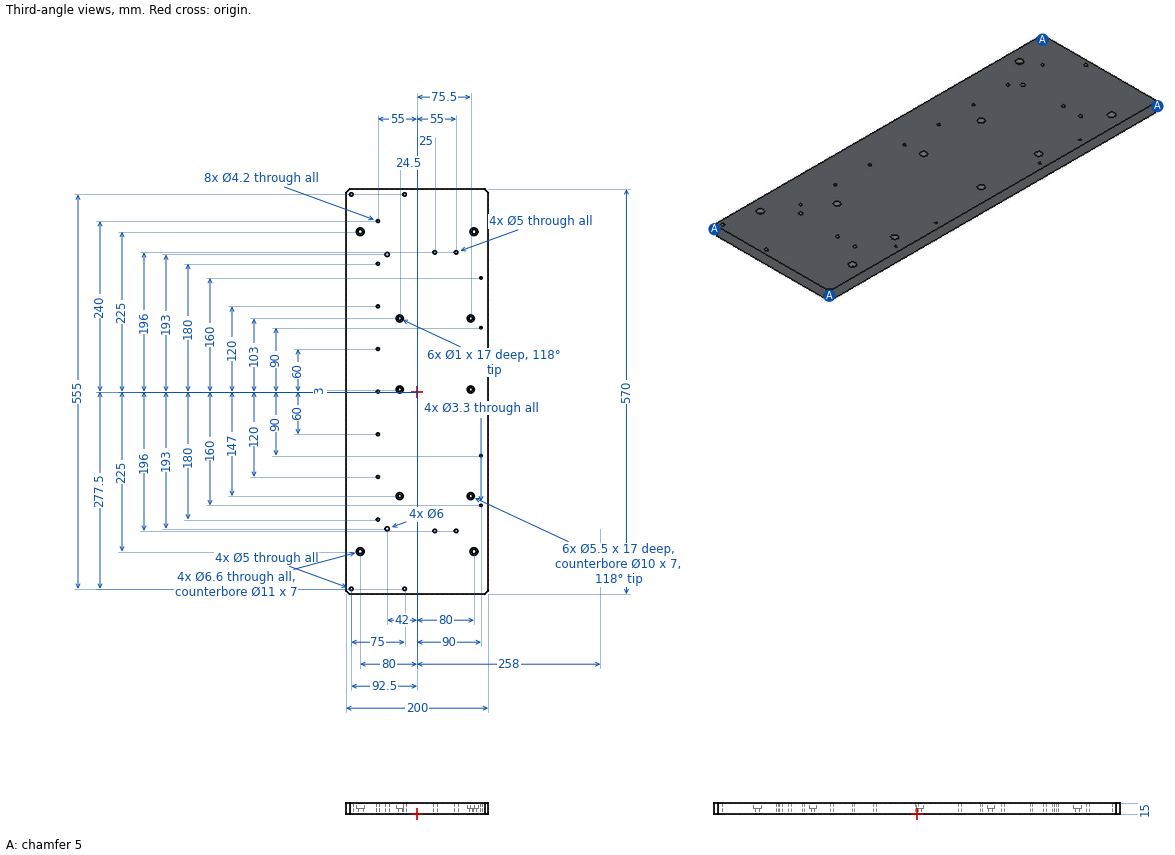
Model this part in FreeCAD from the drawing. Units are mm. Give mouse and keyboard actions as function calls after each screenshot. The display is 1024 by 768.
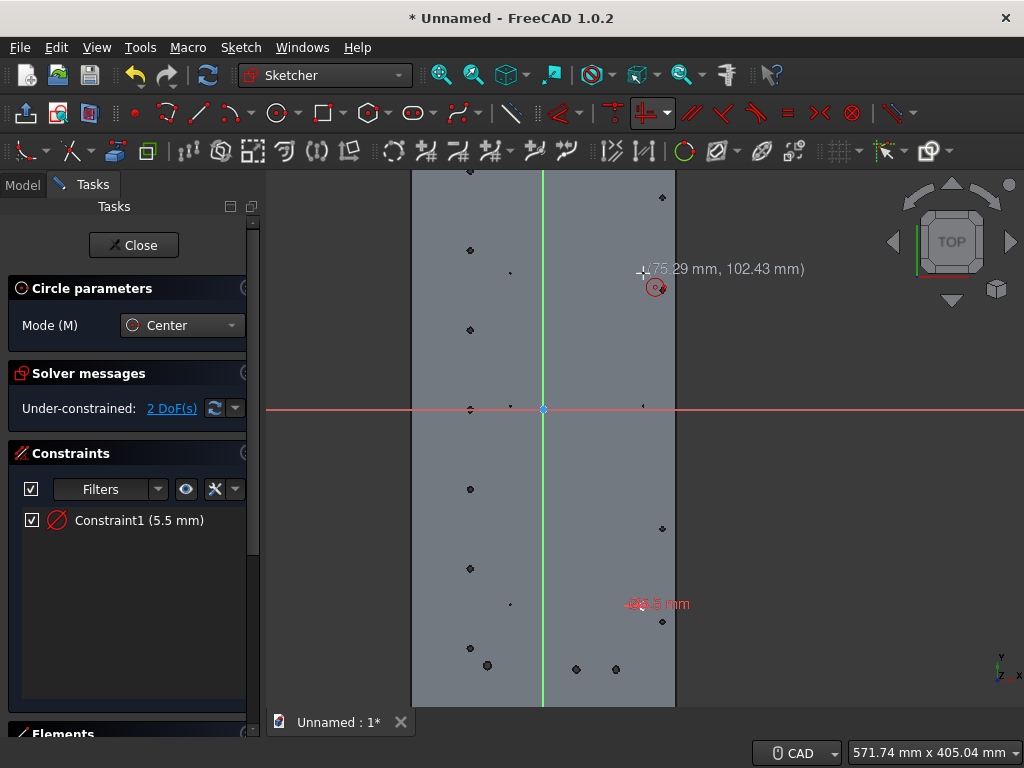
click(643, 273)
move(646, 271)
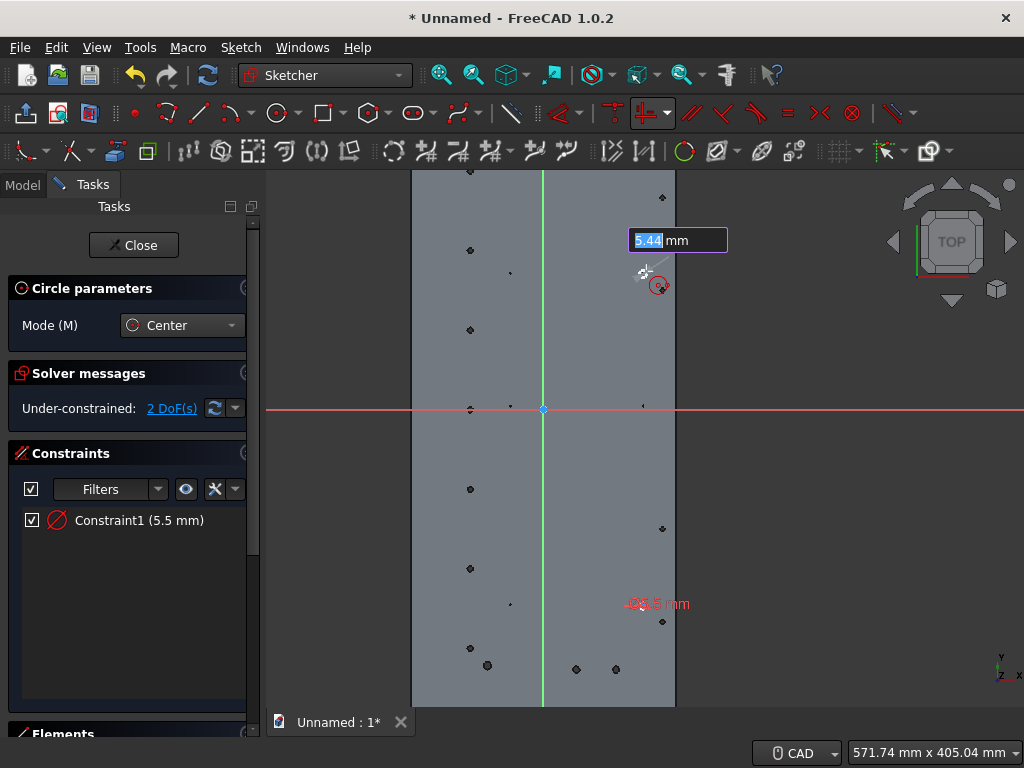
text(5.5)
key(Return)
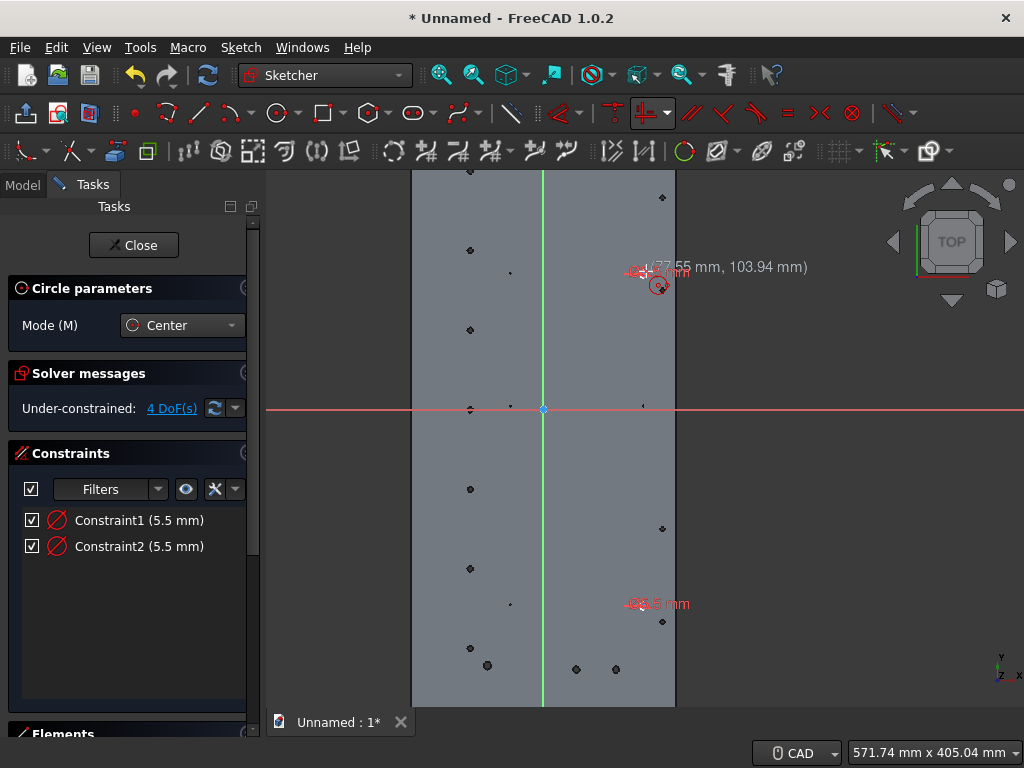
scroll(643, 406, up, 10)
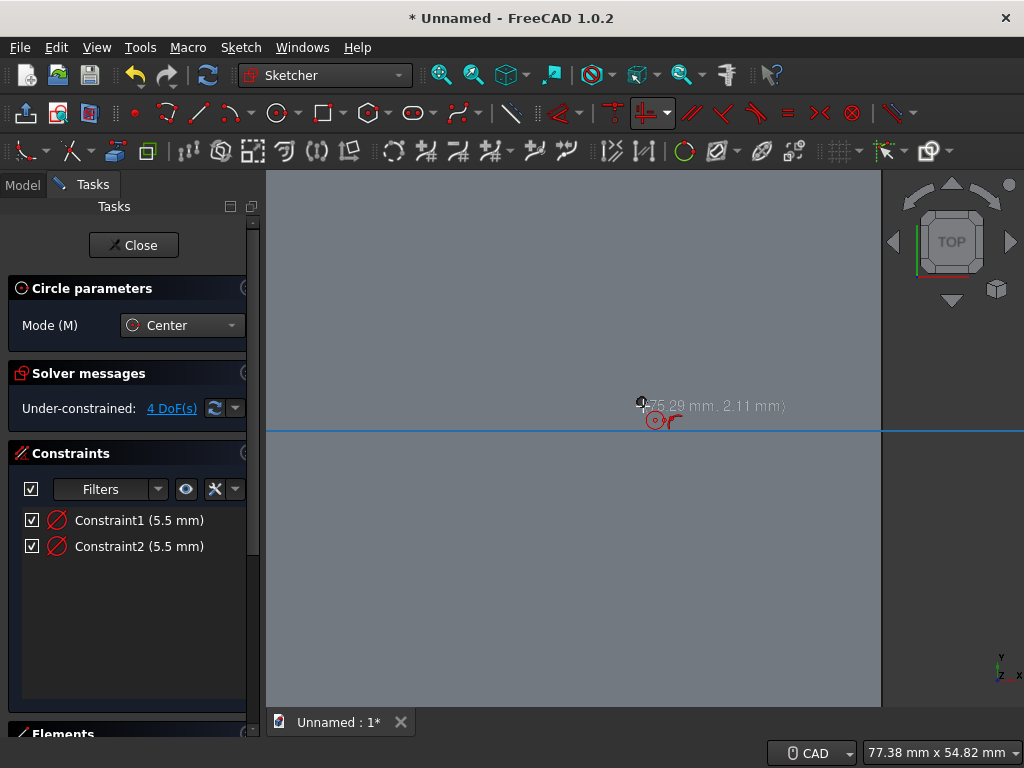
click(642, 402)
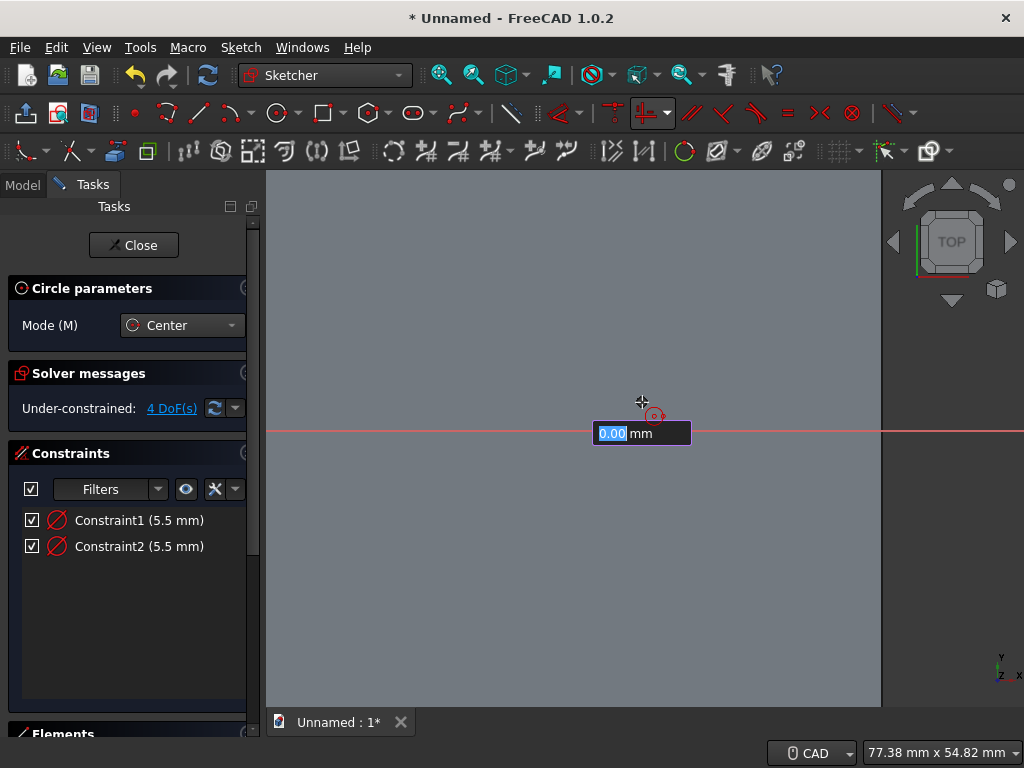
scroll(643, 406, down, 10)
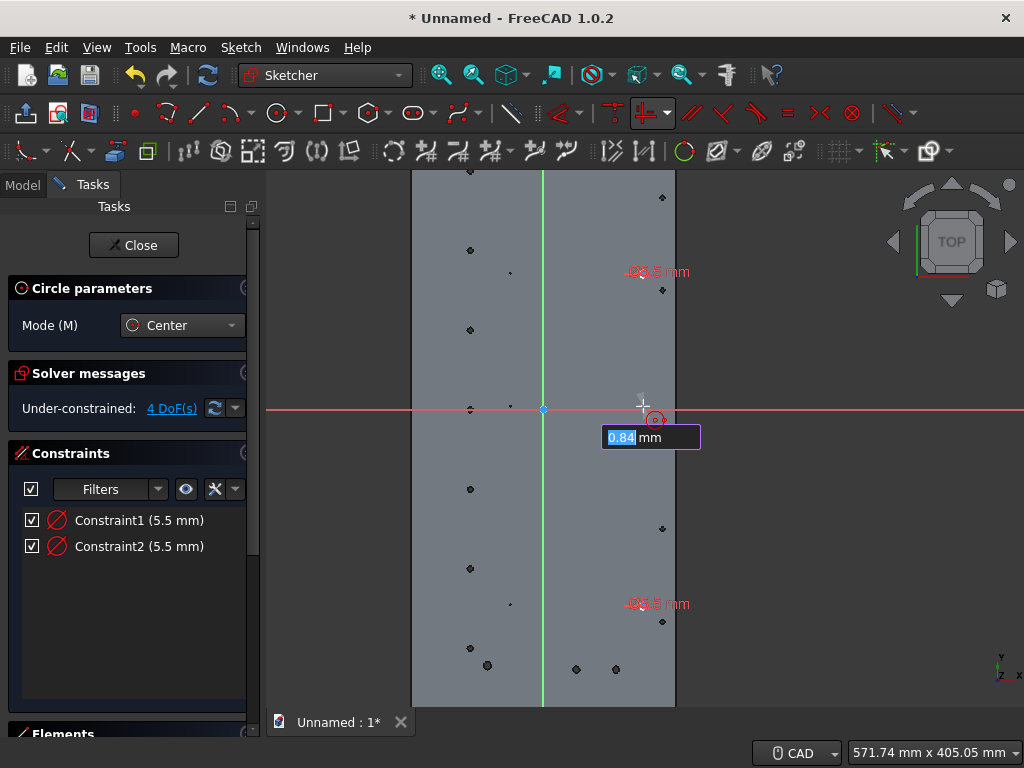
scroll(646, 403, up, 5)
move(645, 403)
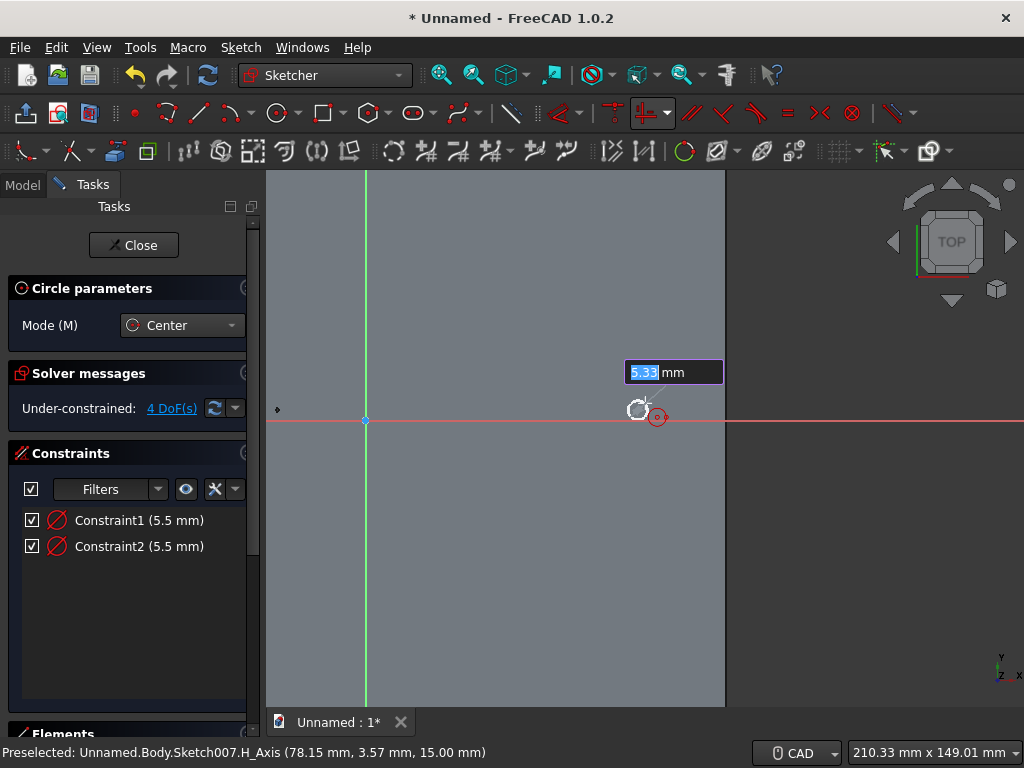
text(5.5)
key(Return)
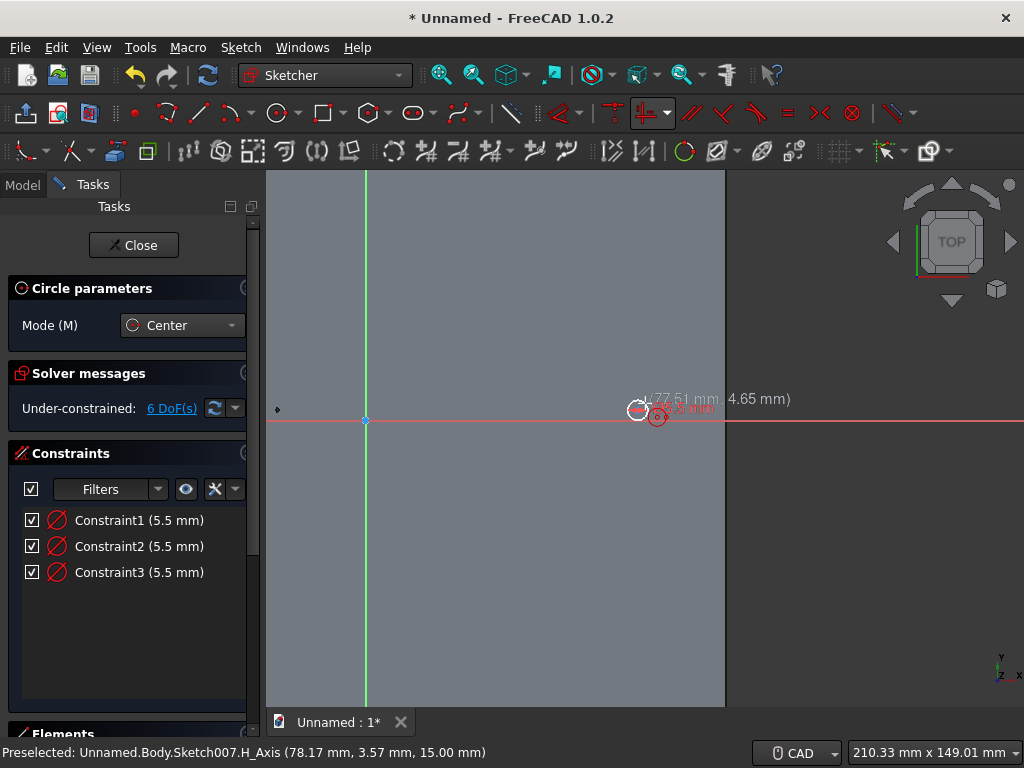
scroll(646, 403, down, 5)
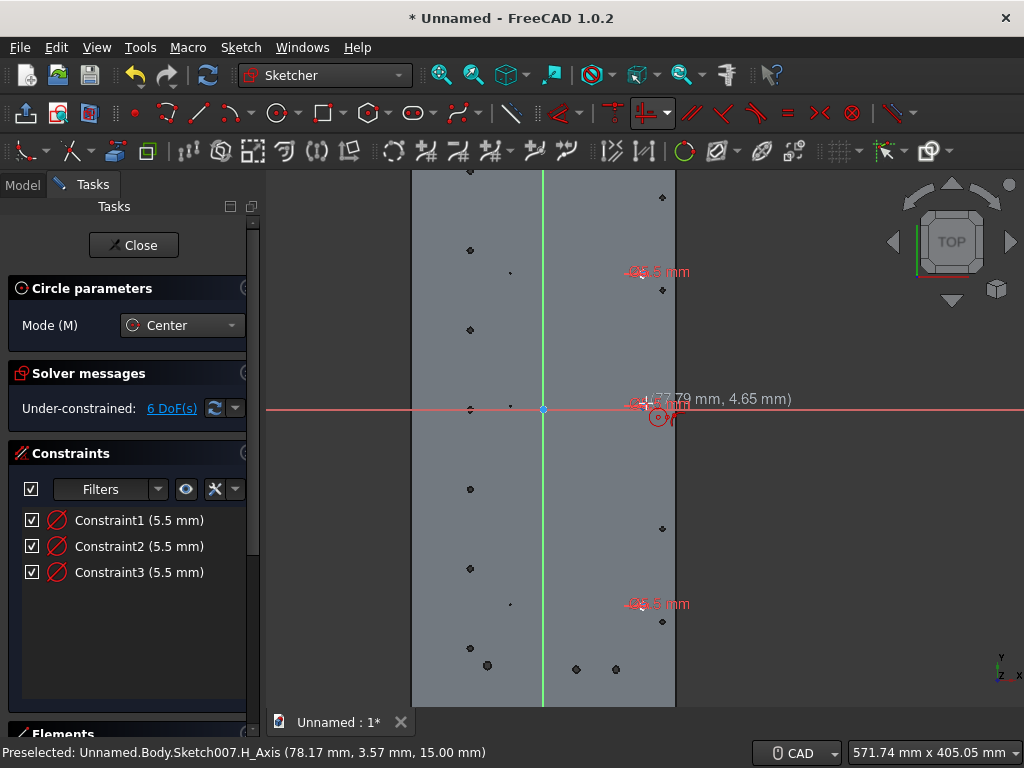
scroll(511, 273, up, 10)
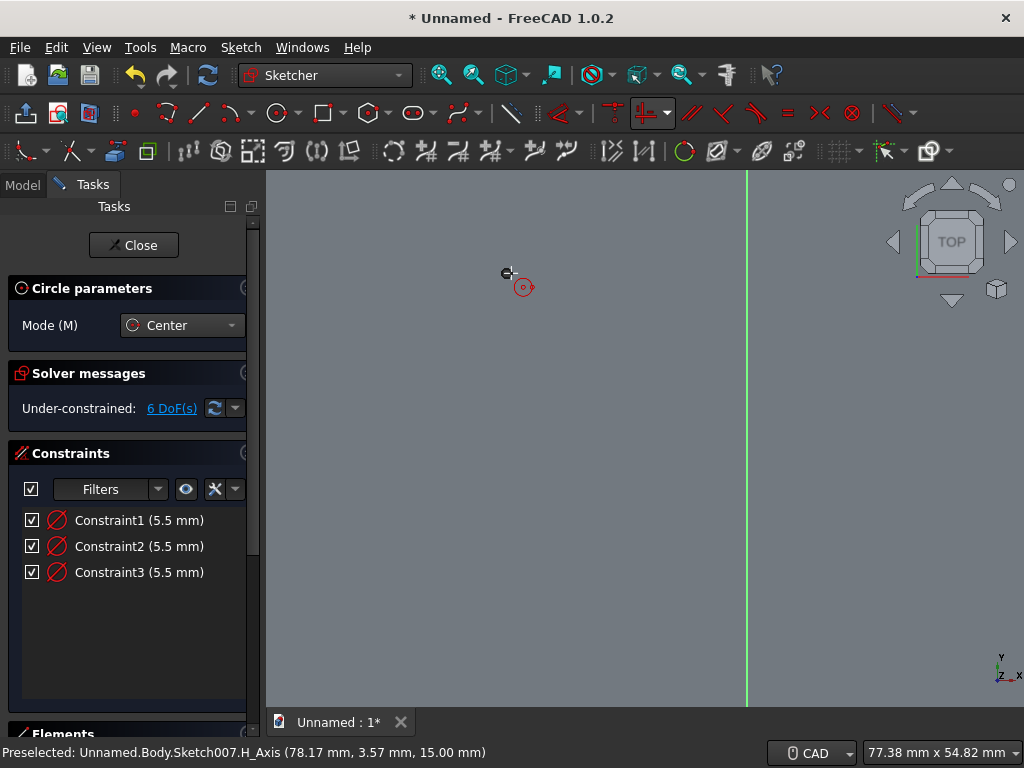
scroll(511, 273, down, 10)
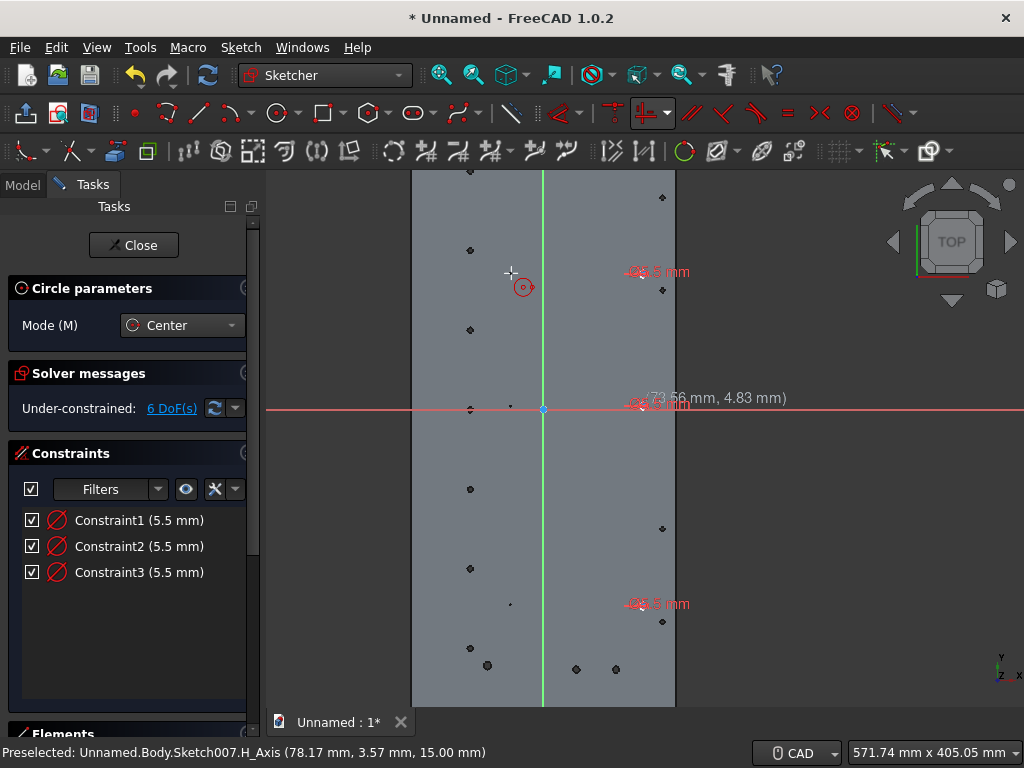
click(511, 273)
move(513, 271)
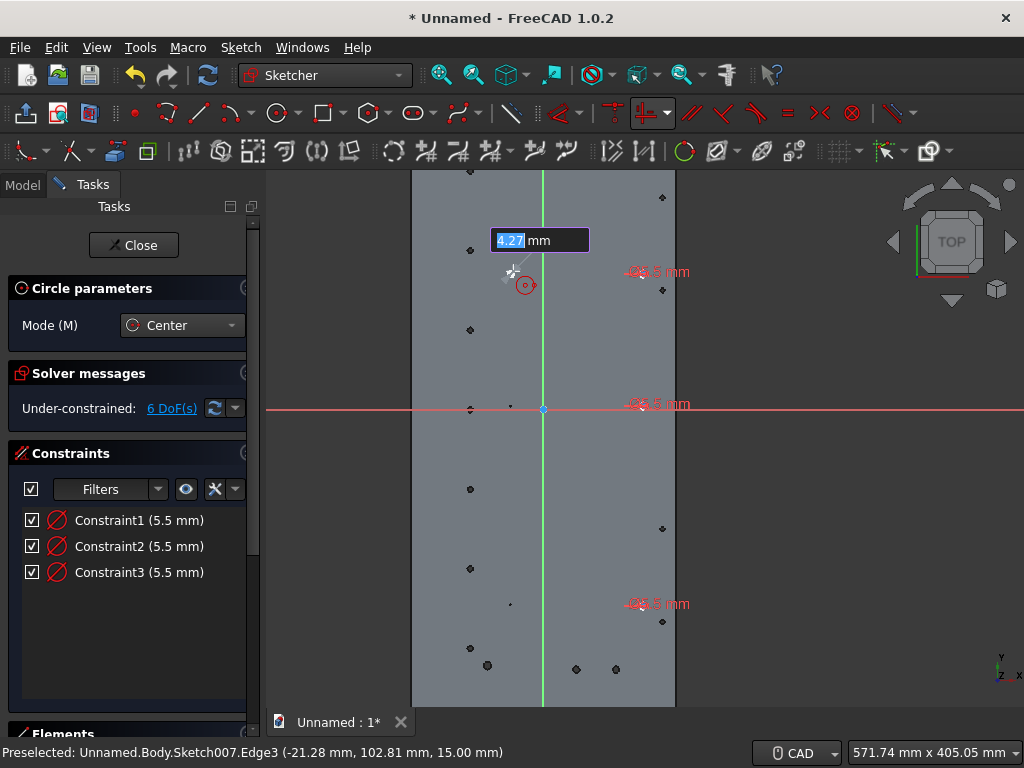
text(5.5)
key(Return)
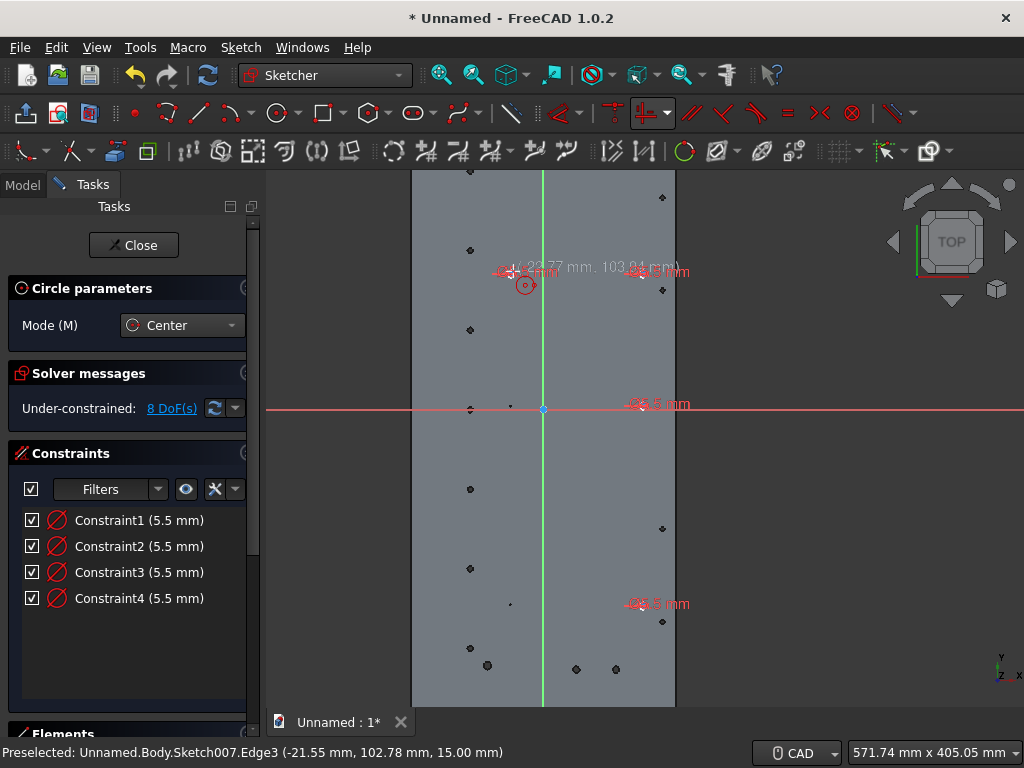
scroll(511, 406, up, 10)